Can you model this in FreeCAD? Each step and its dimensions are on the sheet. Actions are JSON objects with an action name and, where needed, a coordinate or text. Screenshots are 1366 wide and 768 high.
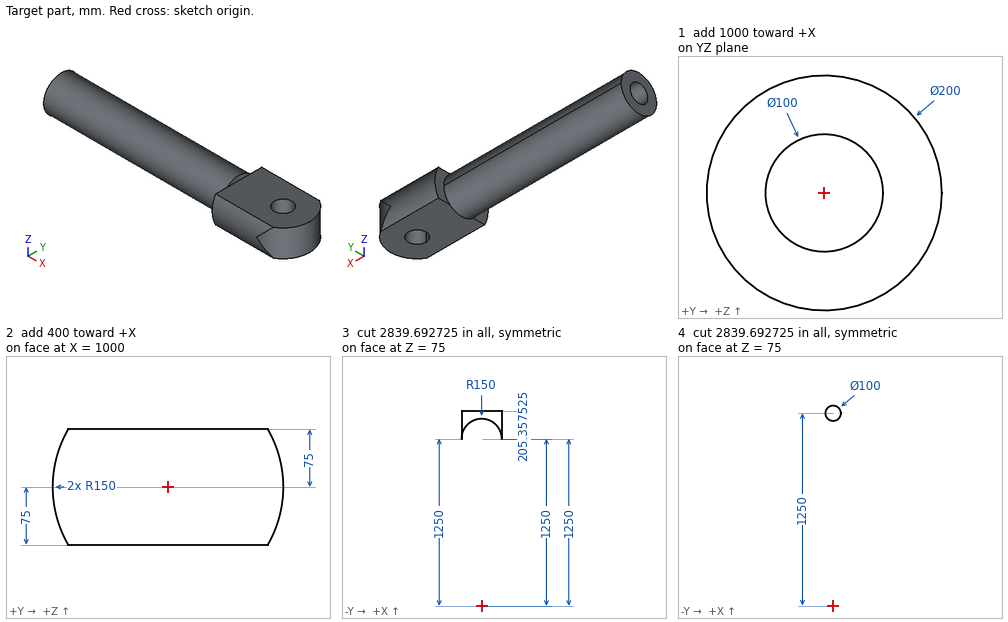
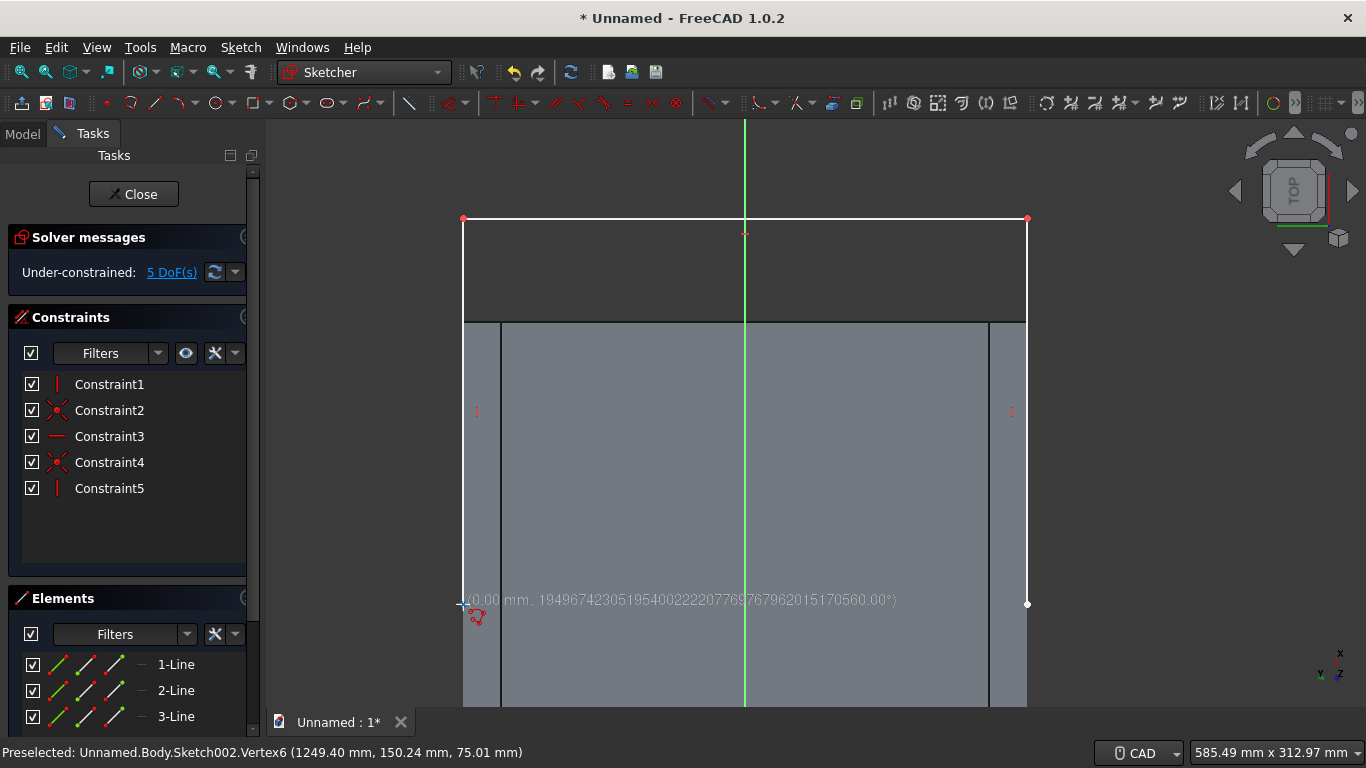
{"action": "left_click", "coordinate": [180, 104]}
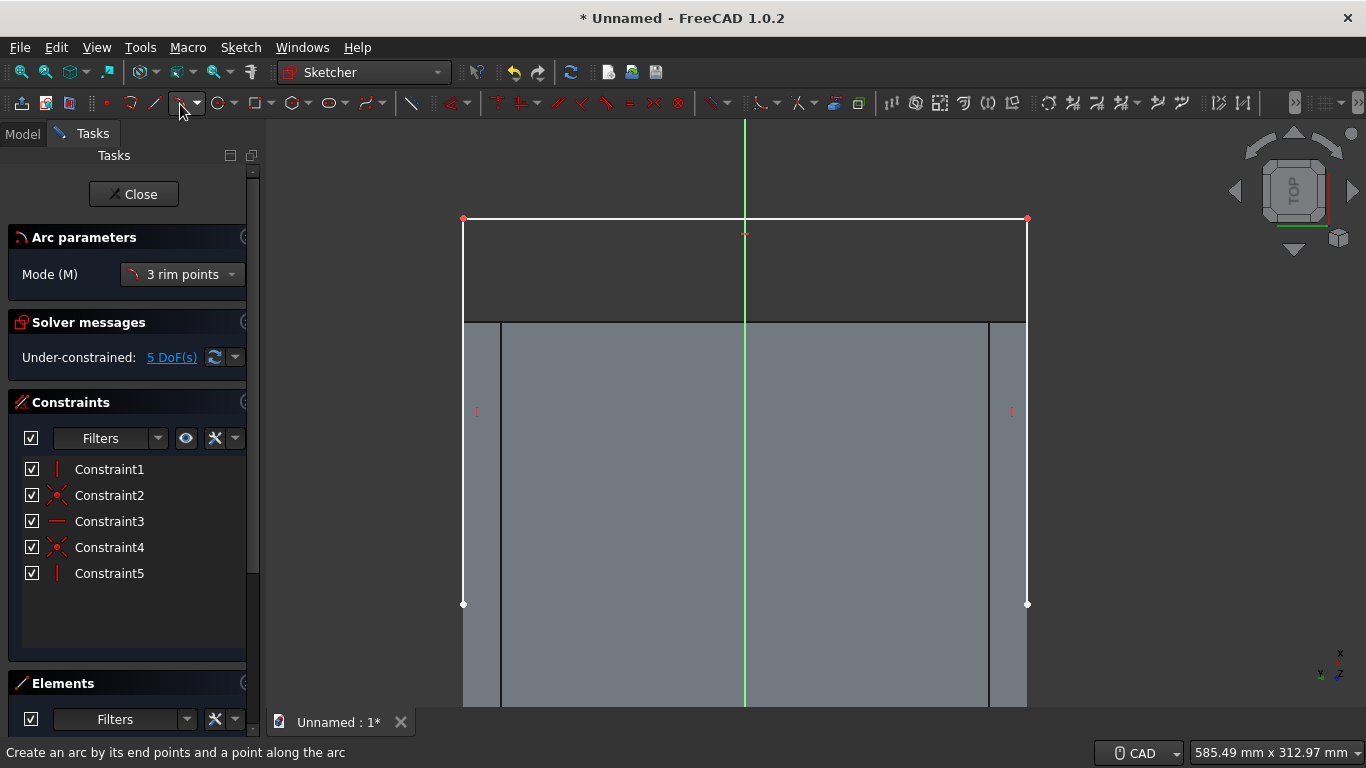
{"action": "left_click", "coordinate": [463, 605]}
{"action": "left_click", "coordinate": [1027, 605]}
{"action": "left_click", "coordinate": [832, 336]}
{"action": "key", "text": "Escape"}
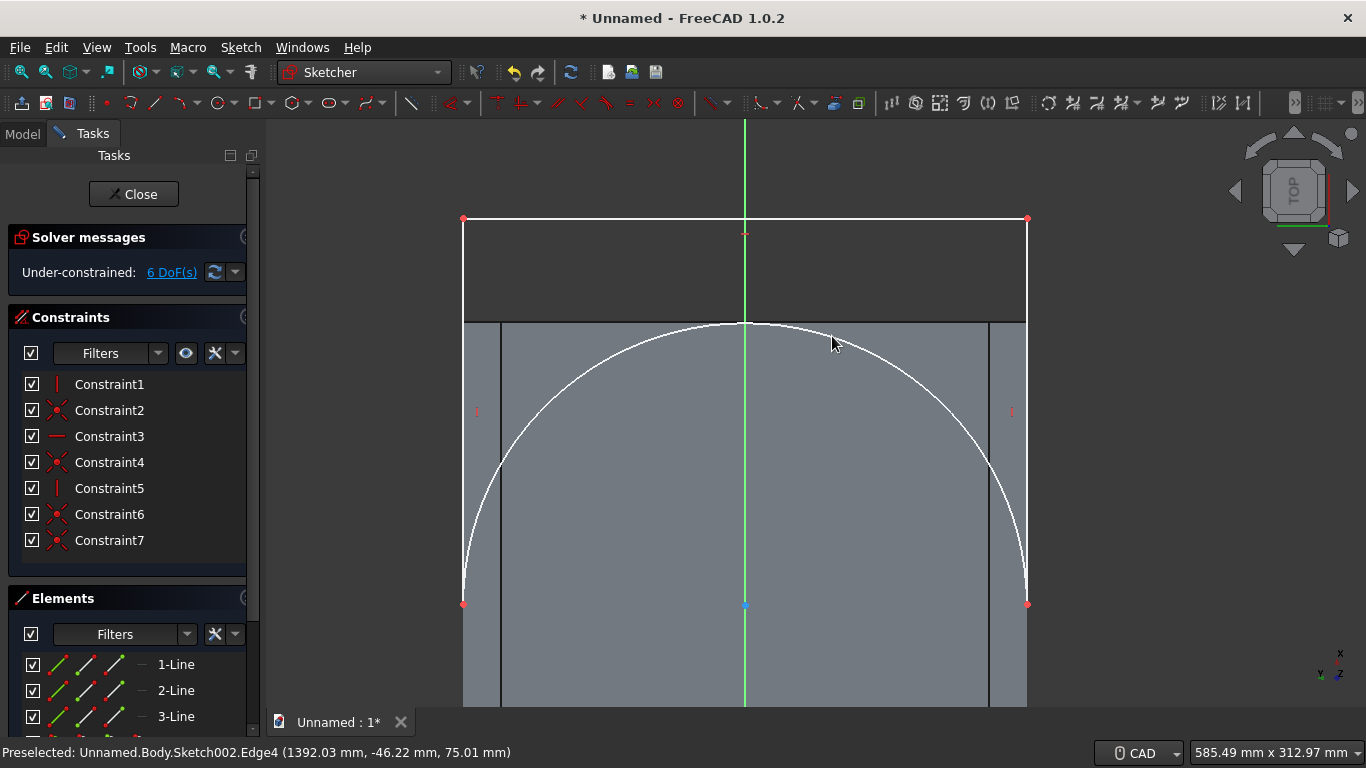
{"action": "left_click", "coordinate": [745, 605]}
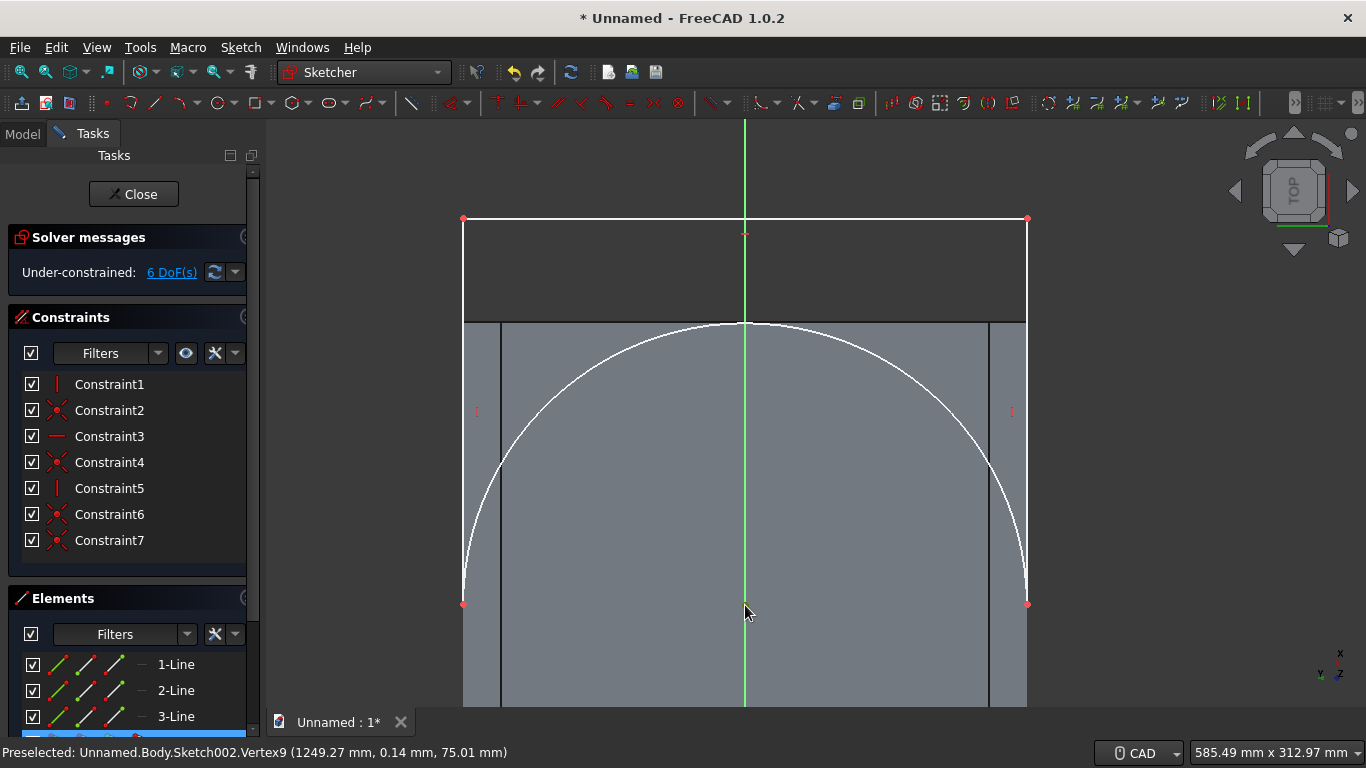
{"action": "left_click", "coordinate": [745, 641]}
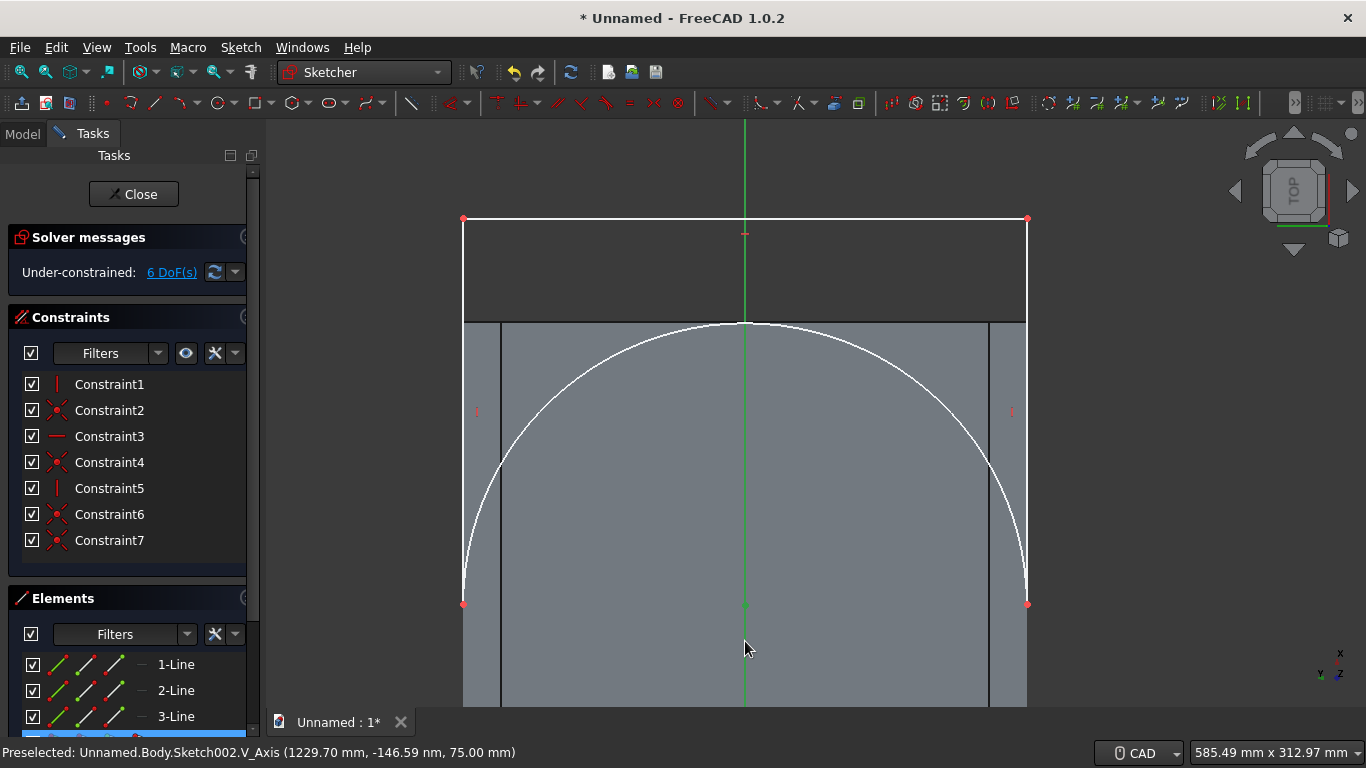
{"action": "left_click", "coordinate": [498, 104]}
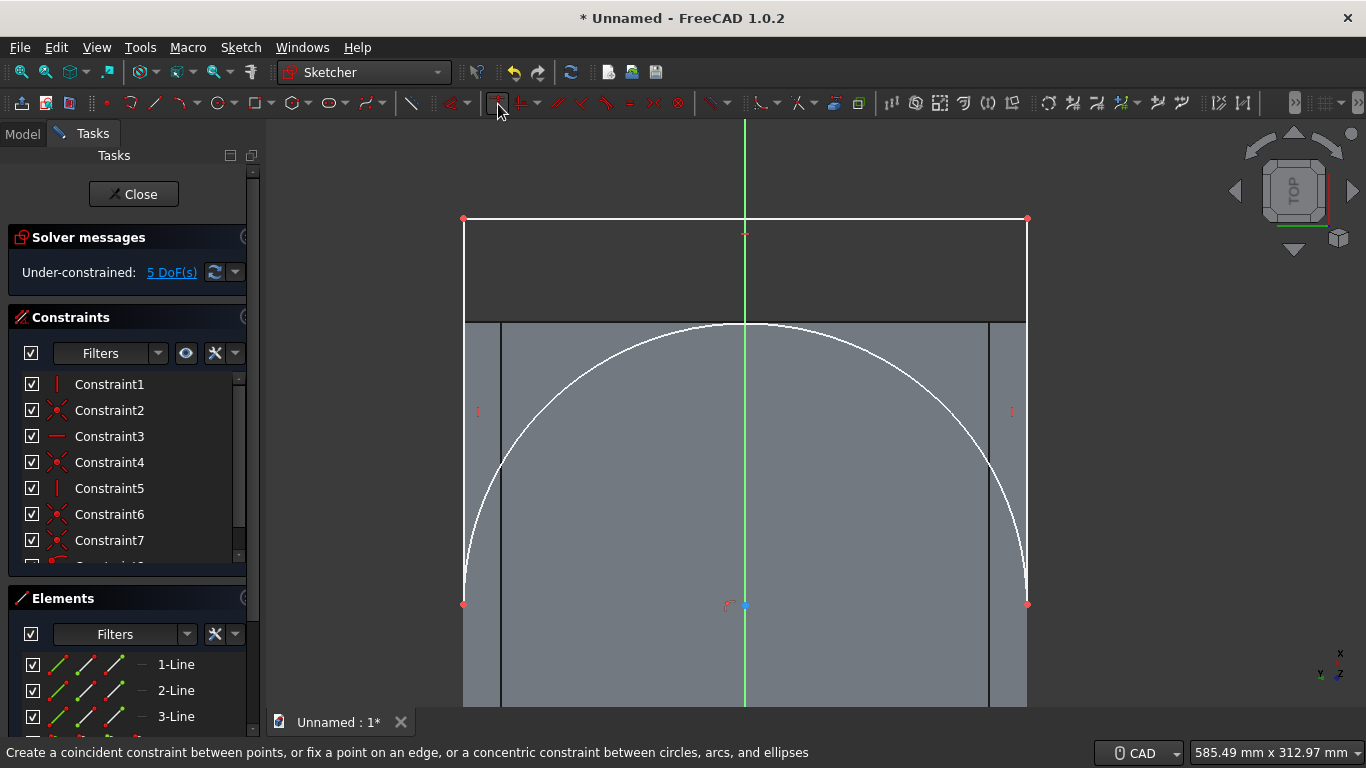
{"action": "left_click", "coordinate": [450, 104]}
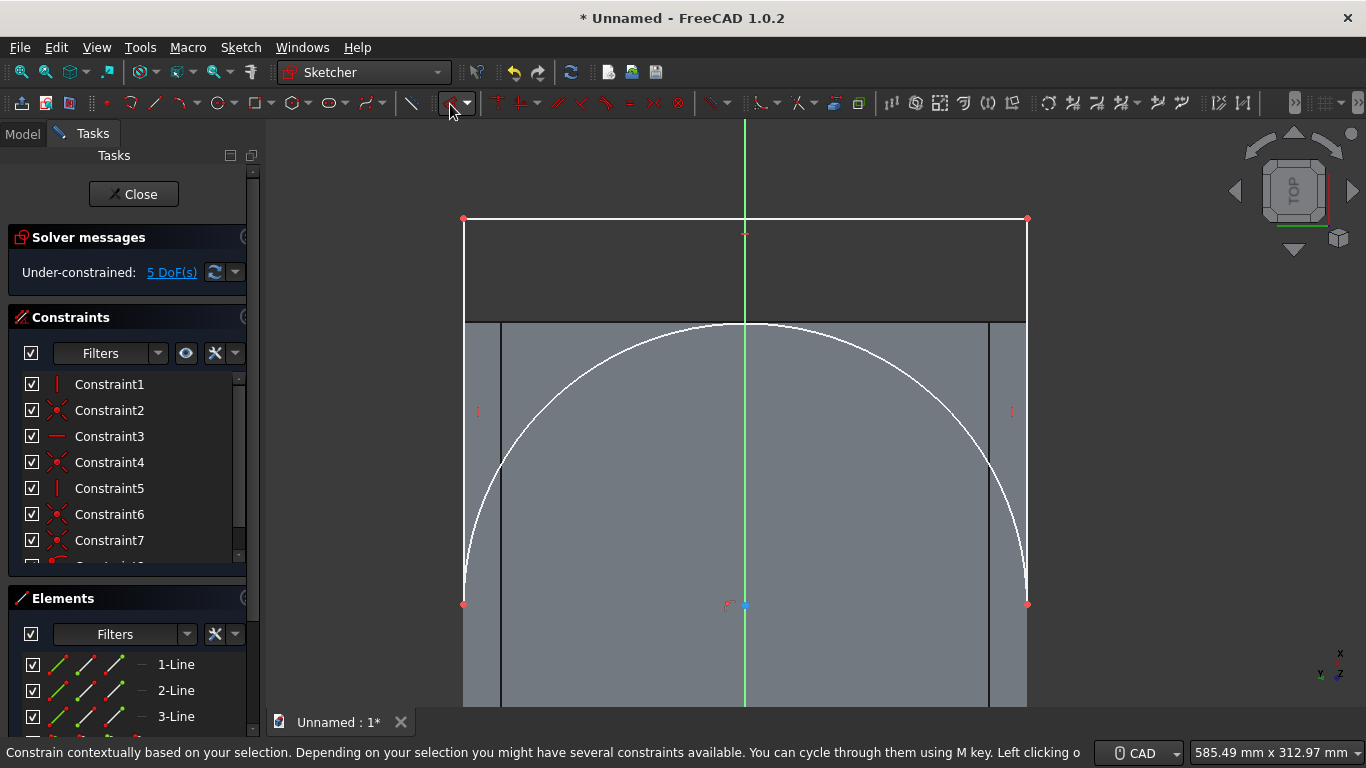
{"action": "left_click", "coordinate": [911, 377]}
{"action": "left_click", "coordinate": [930, 351]}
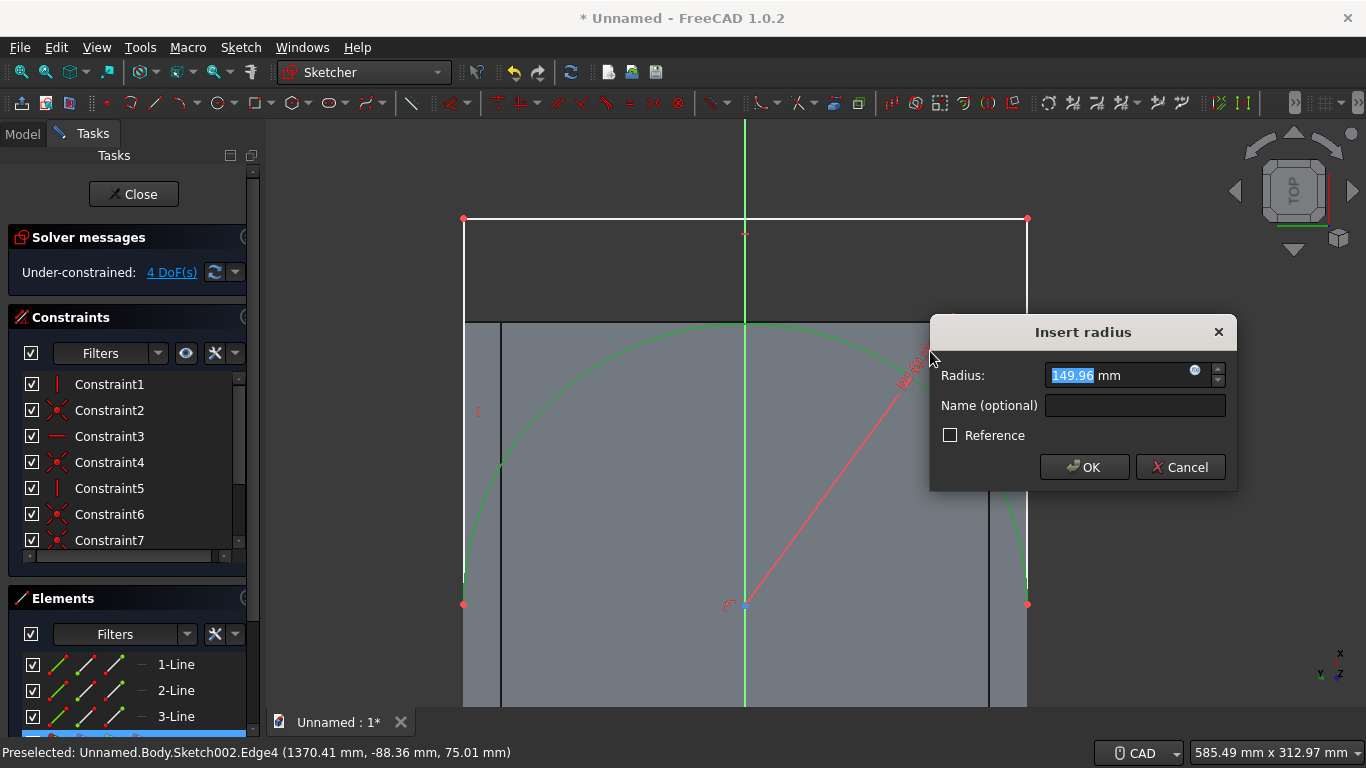
{"action": "type", "text": "150"}
{"action": "key", "text": "Return"}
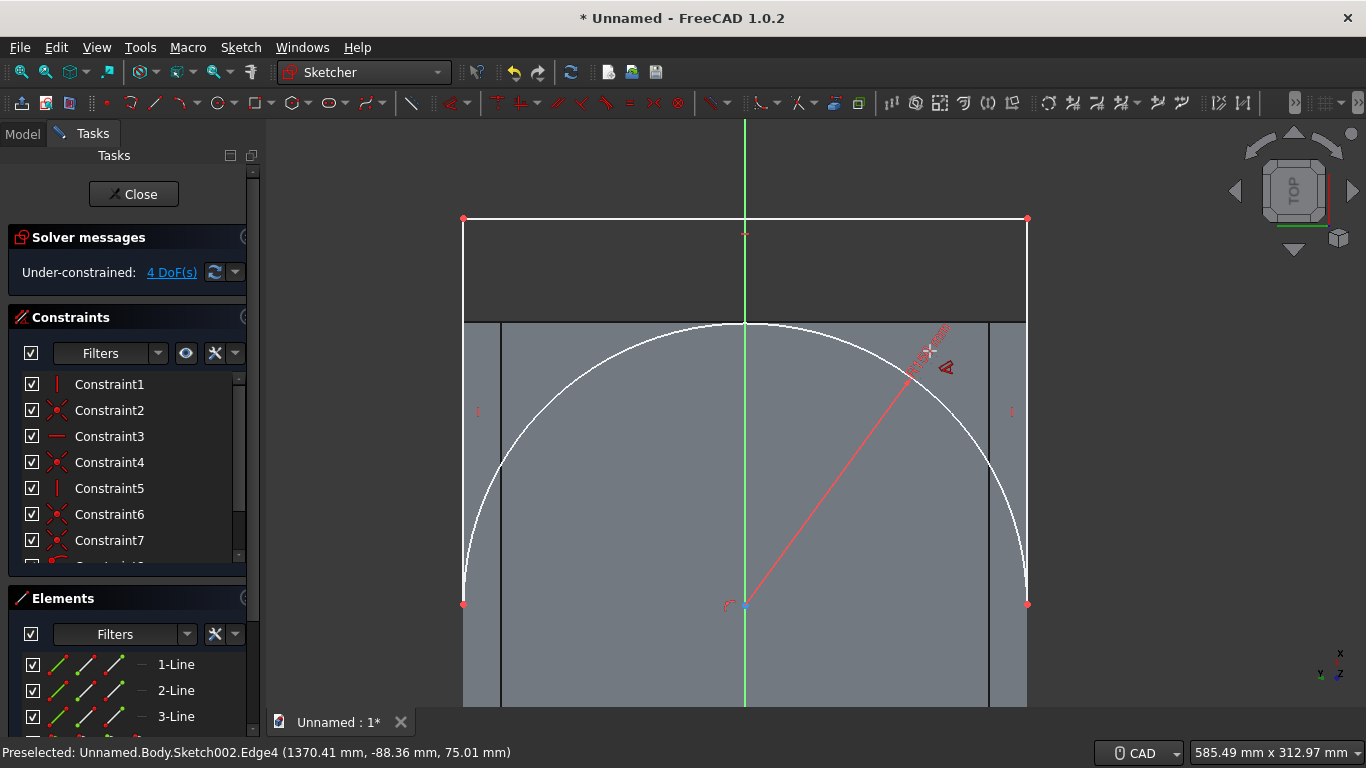
{"action": "left_click", "coordinate": [1027, 605]}
{"action": "left_click", "coordinate": [1061, 642]}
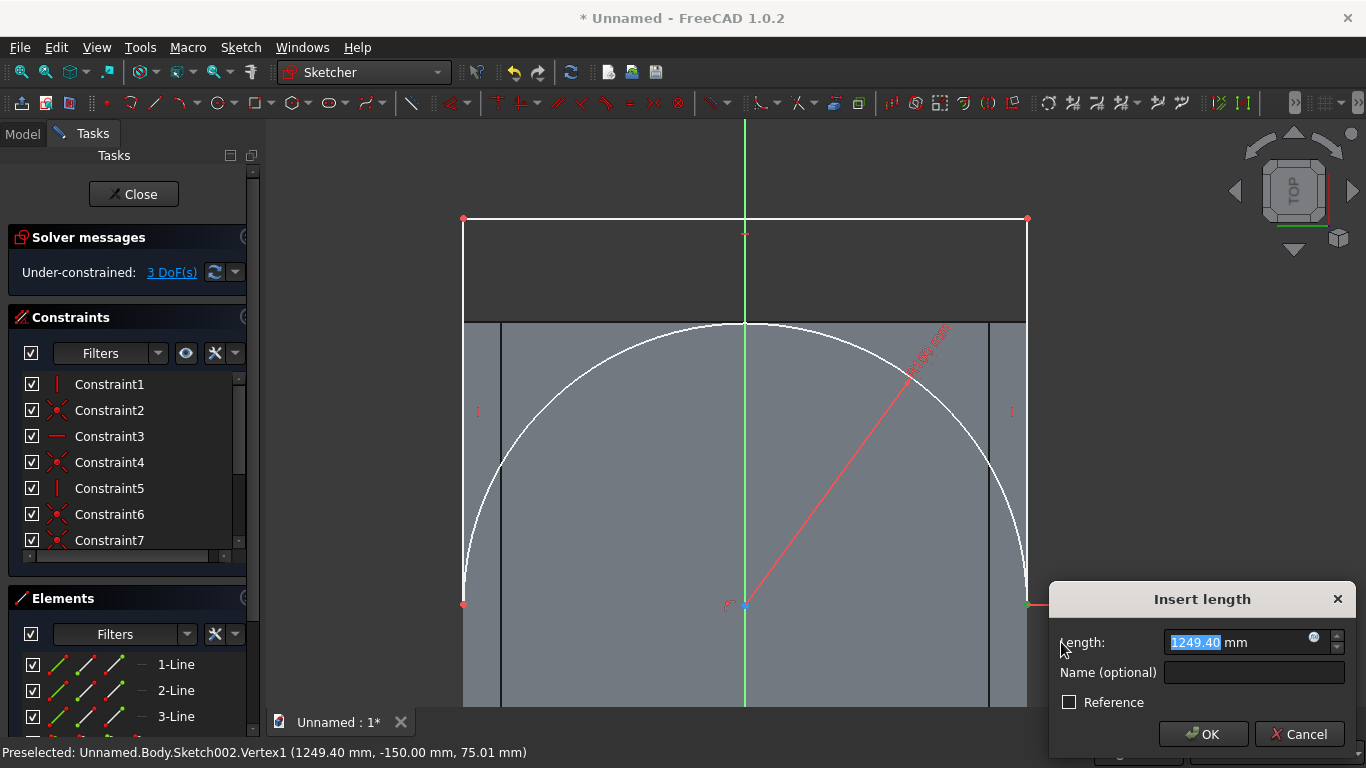
{"action": "type", "text": "1250"}
{"action": "key", "text": "Return"}